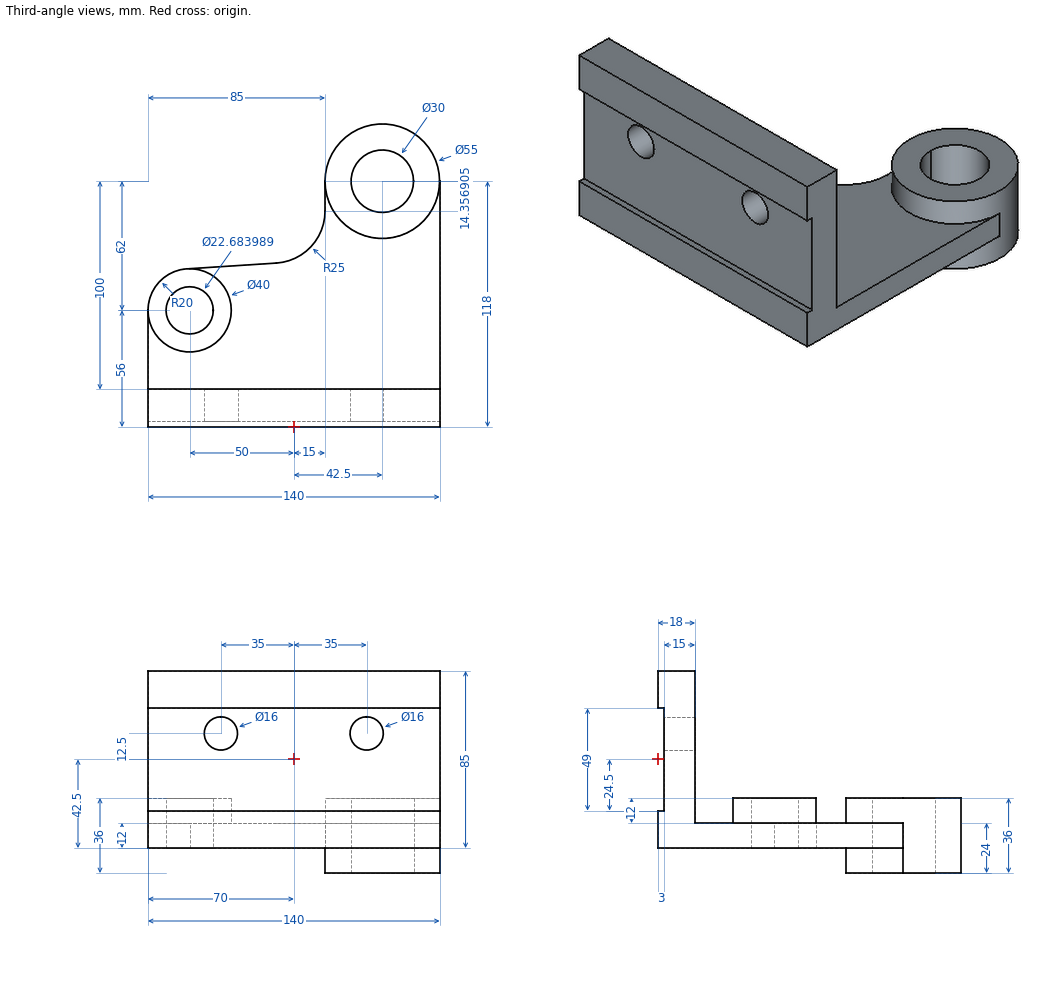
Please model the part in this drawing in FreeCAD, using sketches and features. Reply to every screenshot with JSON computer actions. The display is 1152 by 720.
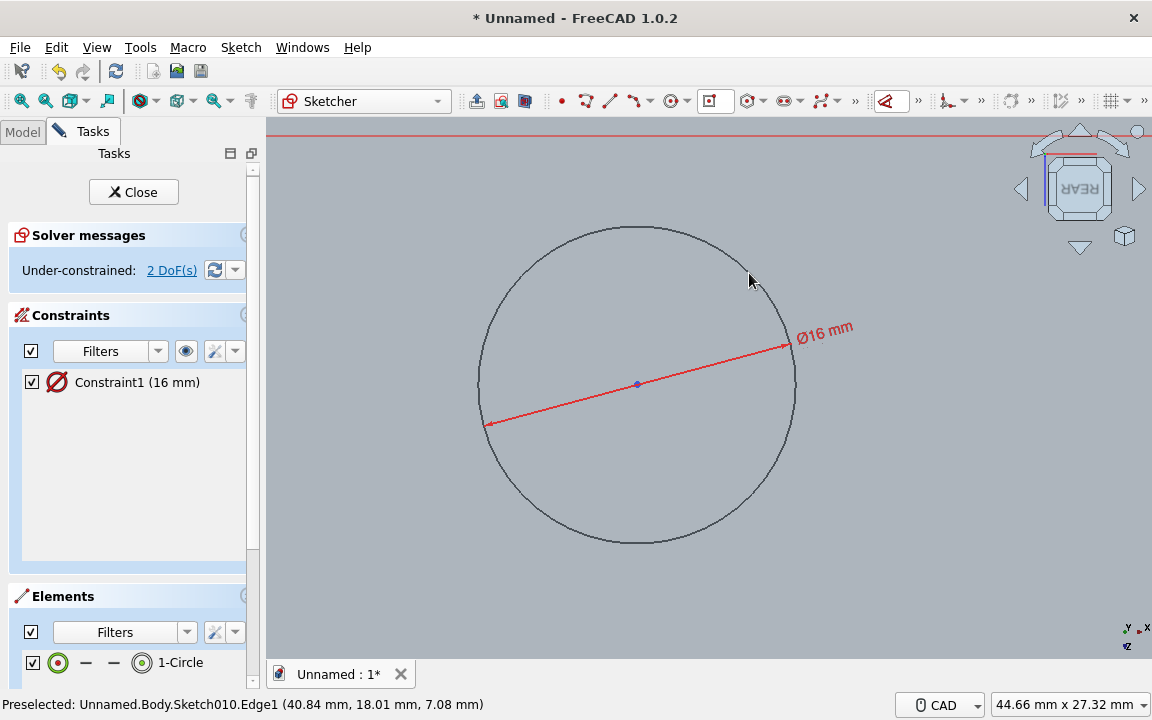
{"action": "left_click", "coordinate": [637, 385]}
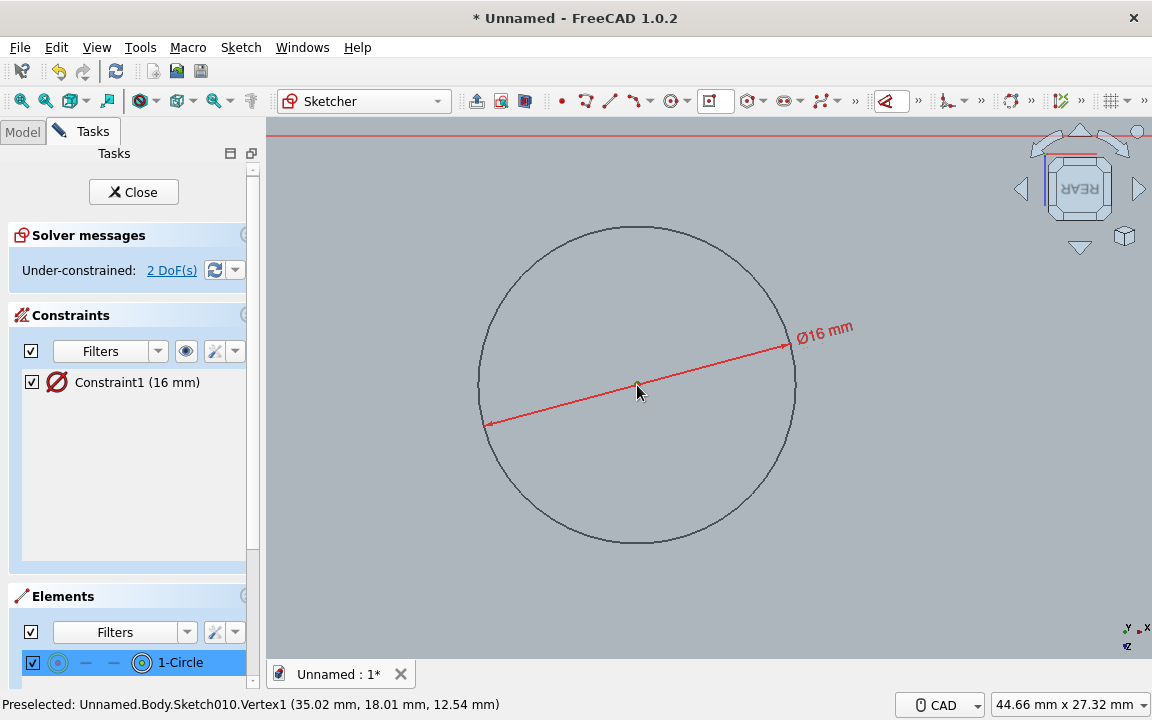
{"action": "key", "text": "l"}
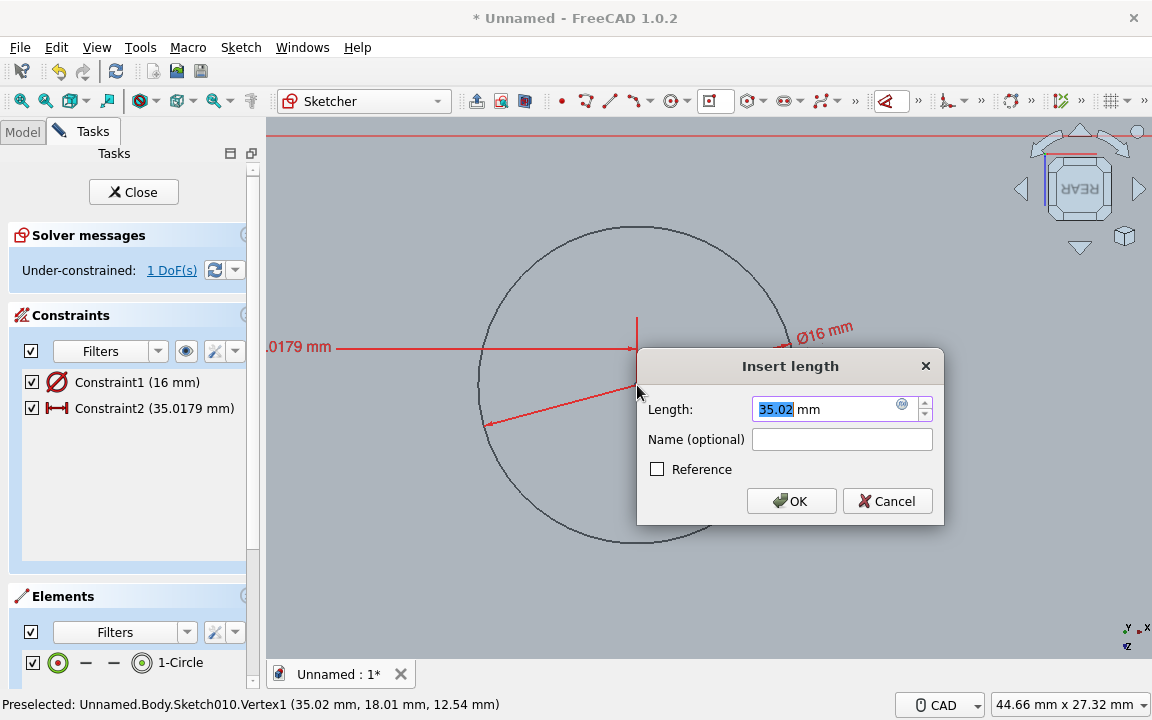
{"action": "type", "text": "35"}
{"action": "key", "text": "Return"}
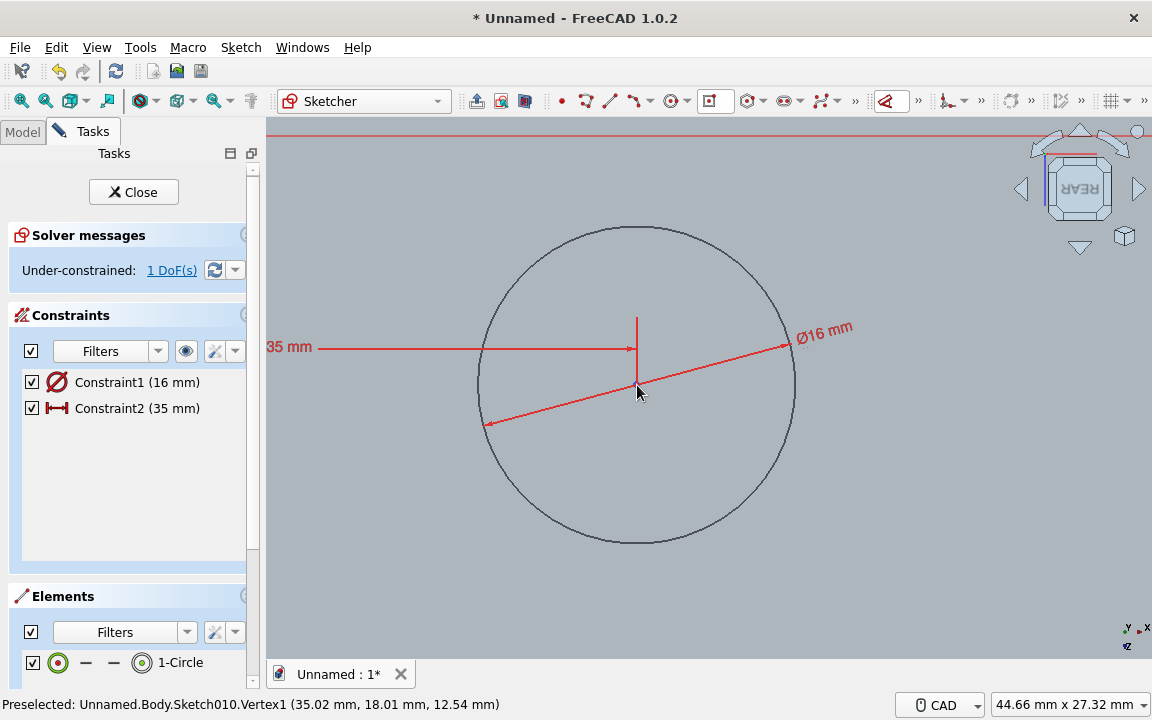
{"action": "left_click", "coordinate": [637, 385]}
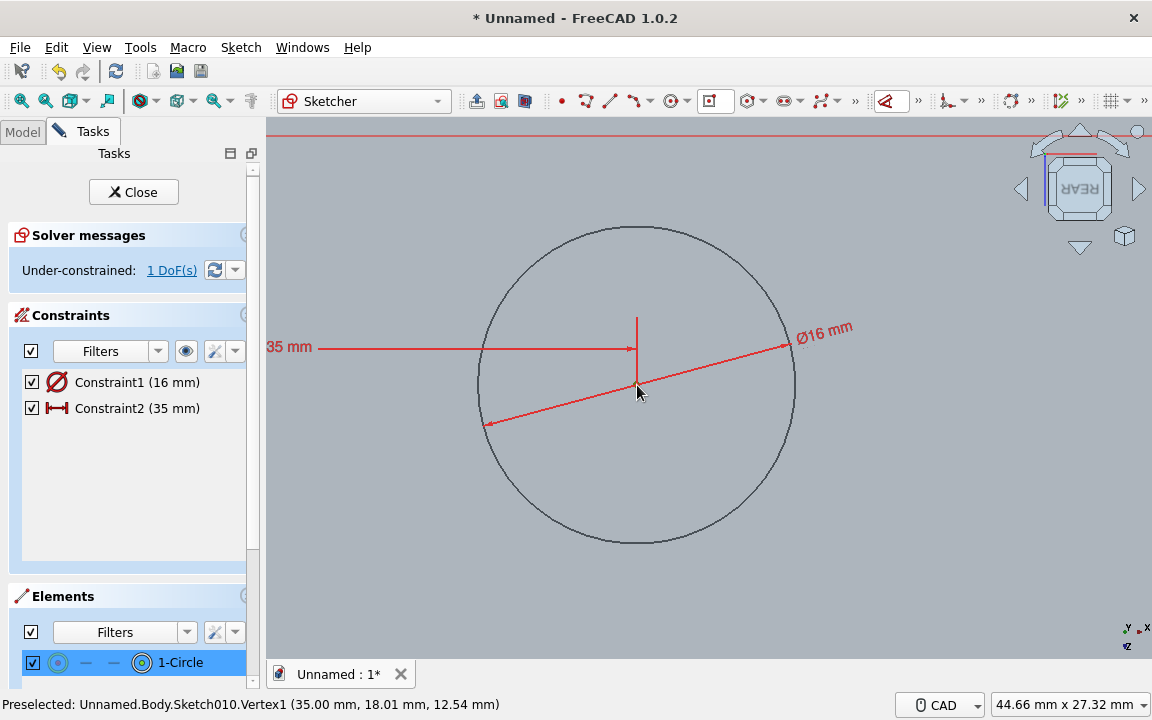
{"action": "key", "text": "i"}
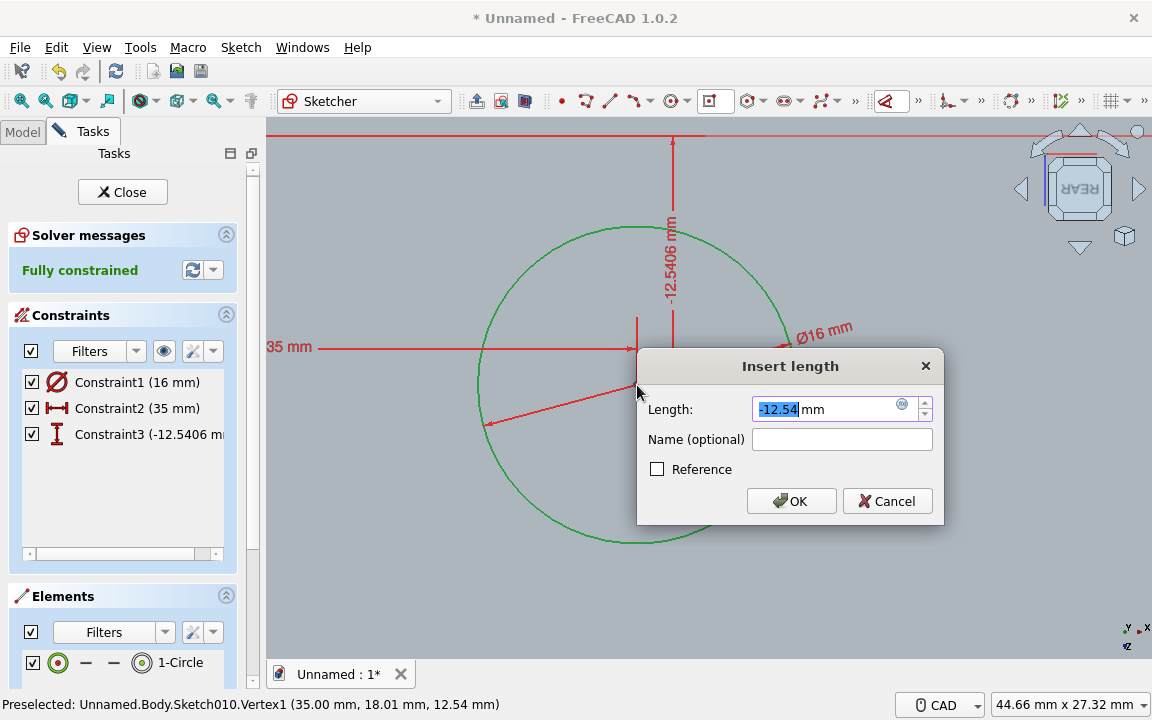
{"action": "type", "text": "-12.5"}
{"action": "key", "text": "Return"}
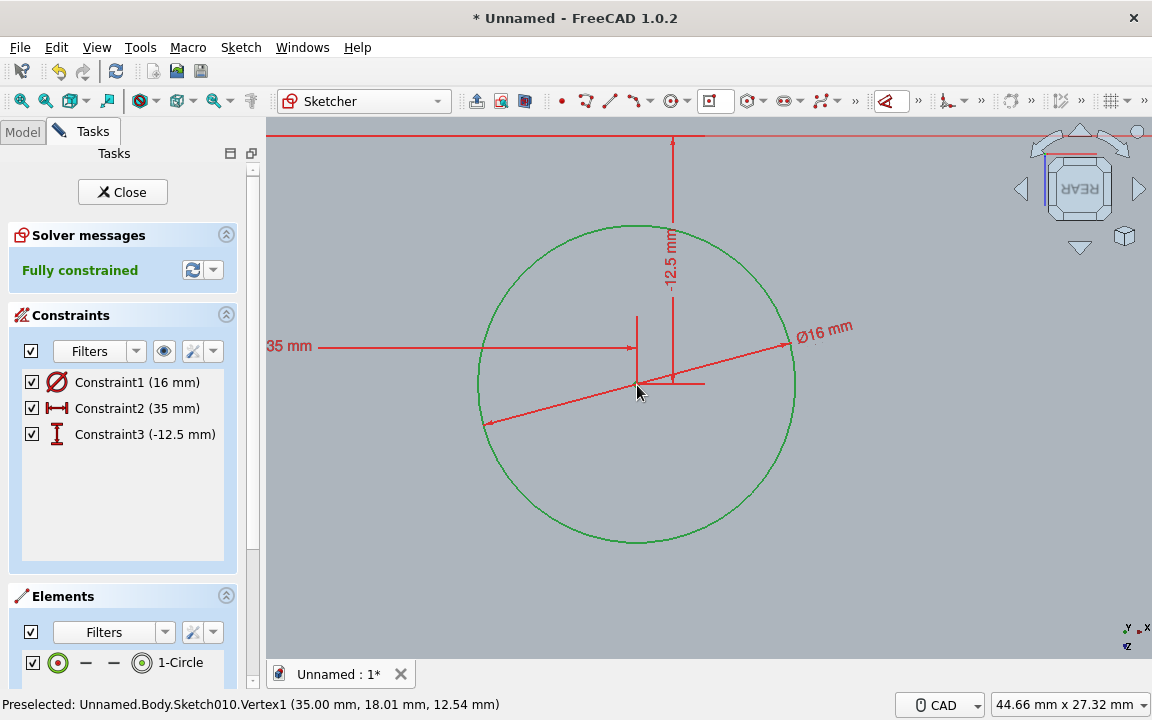
{"action": "left_click", "coordinate": [123, 192]}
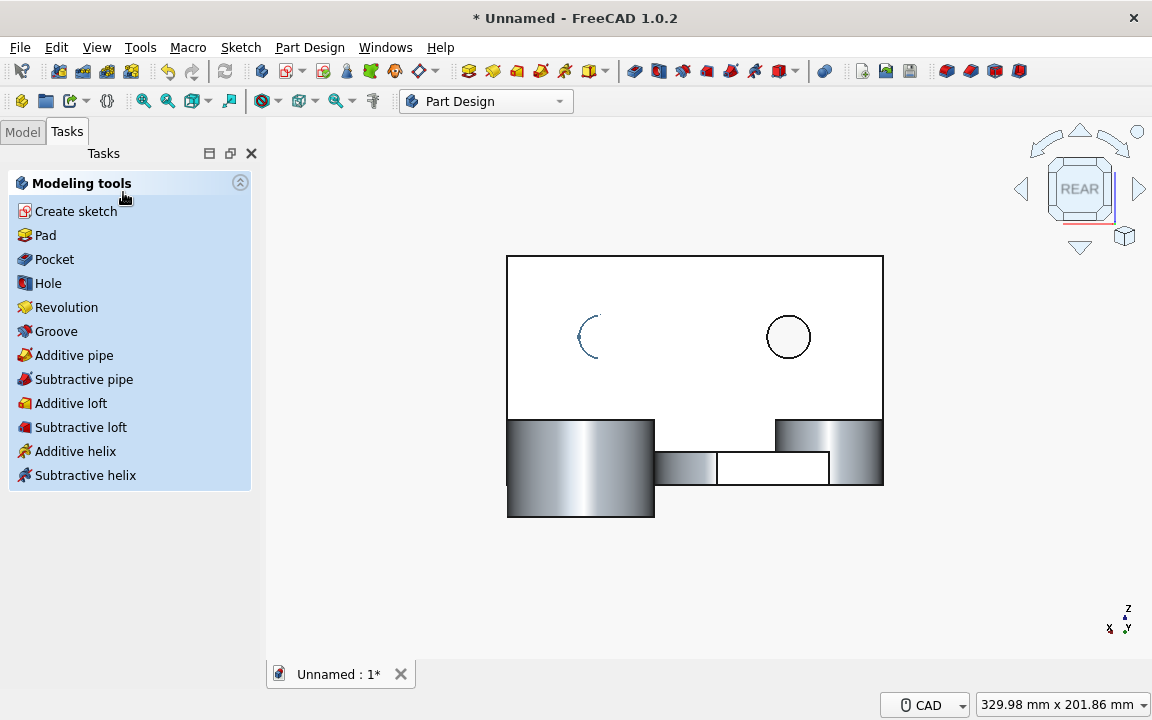
{"action": "left_click", "coordinate": [636, 72]}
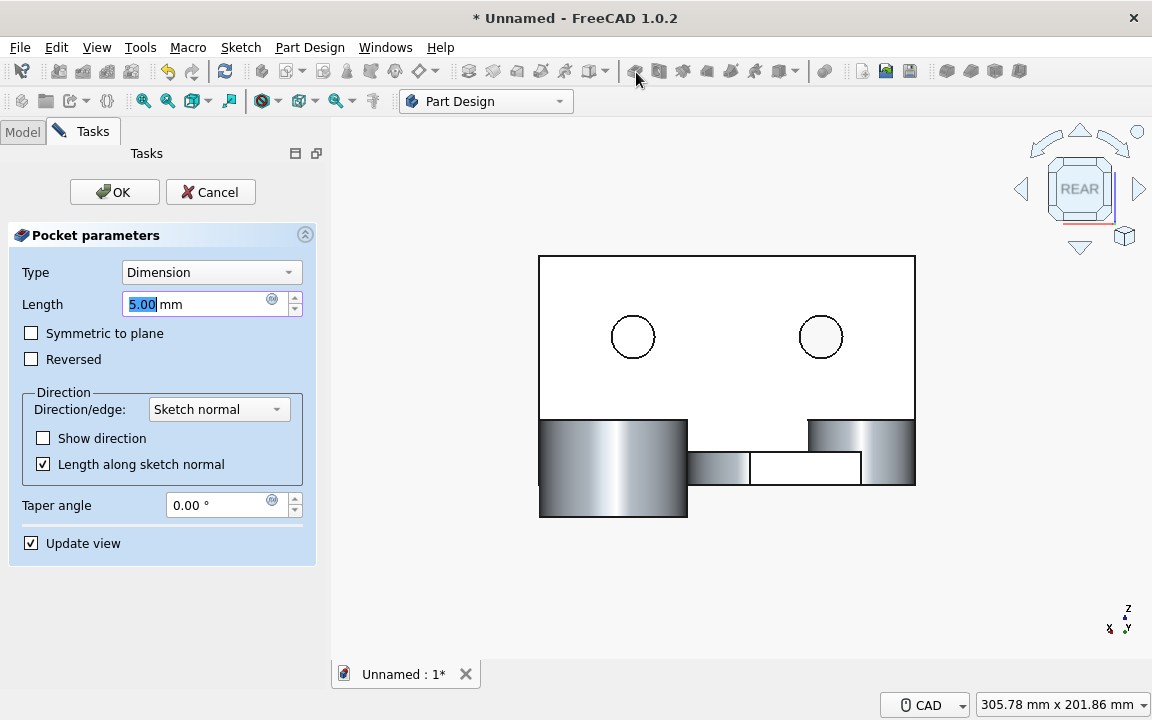
{"action": "type", "text": "15"}
{"action": "key", "text": "Tab"}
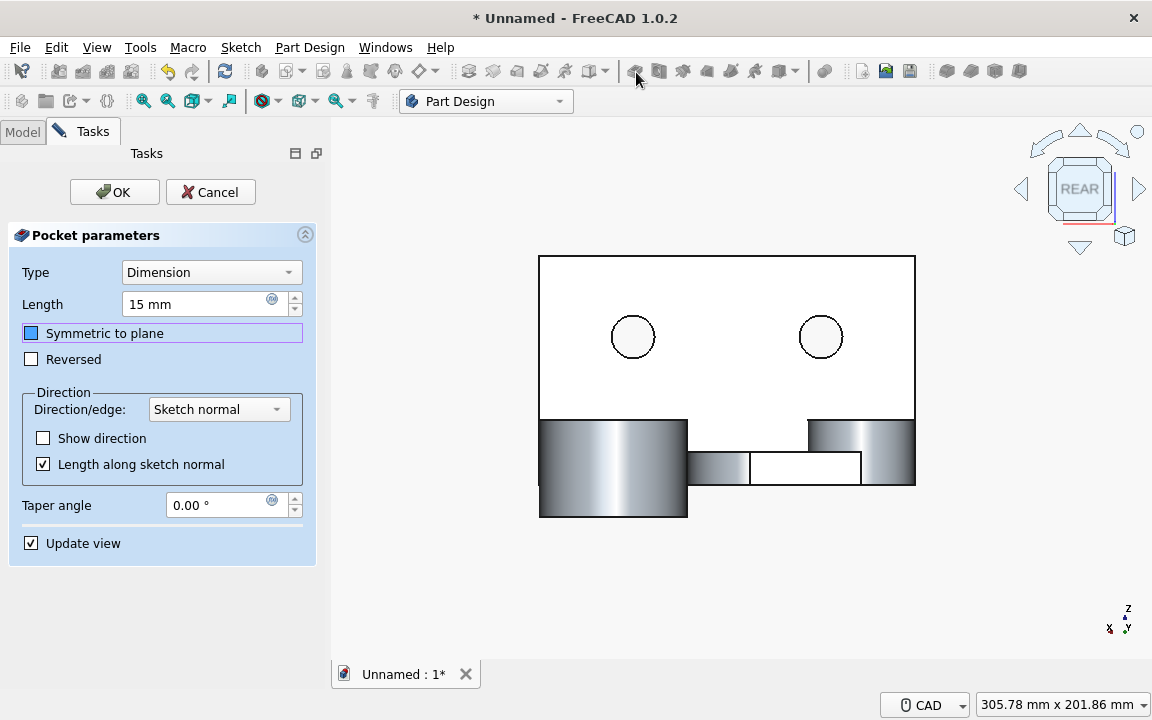
{"action": "left_click", "coordinate": [115, 192]}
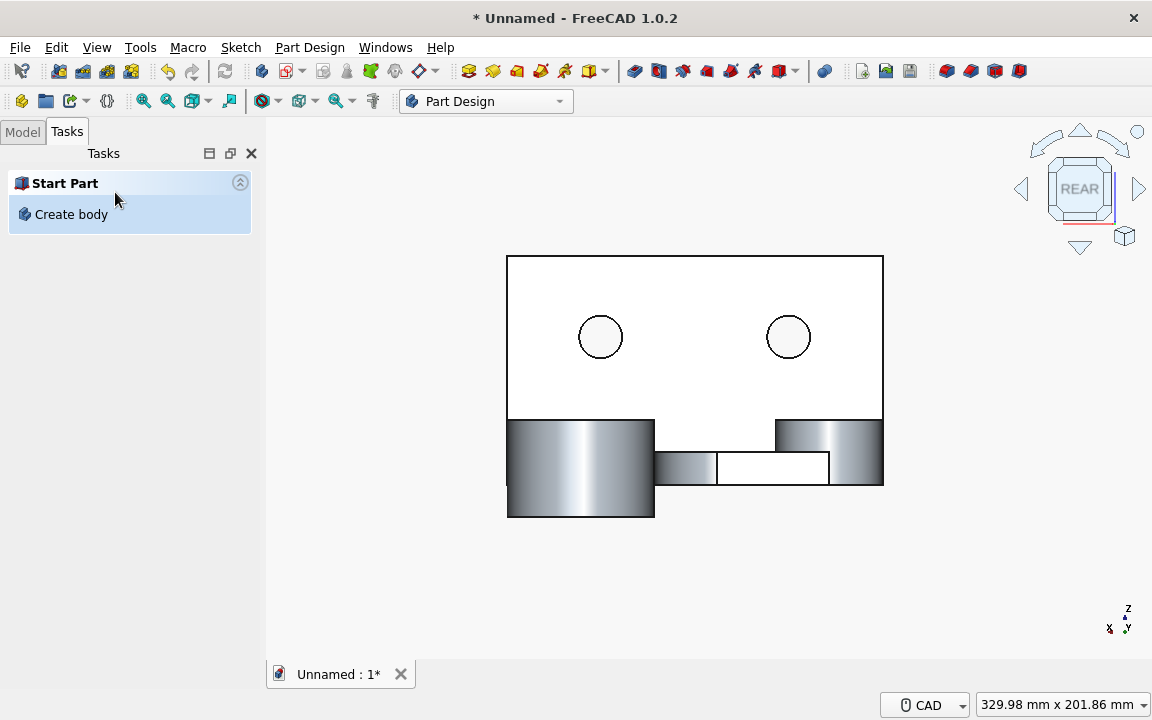
{"action": "key", "text": "0"}